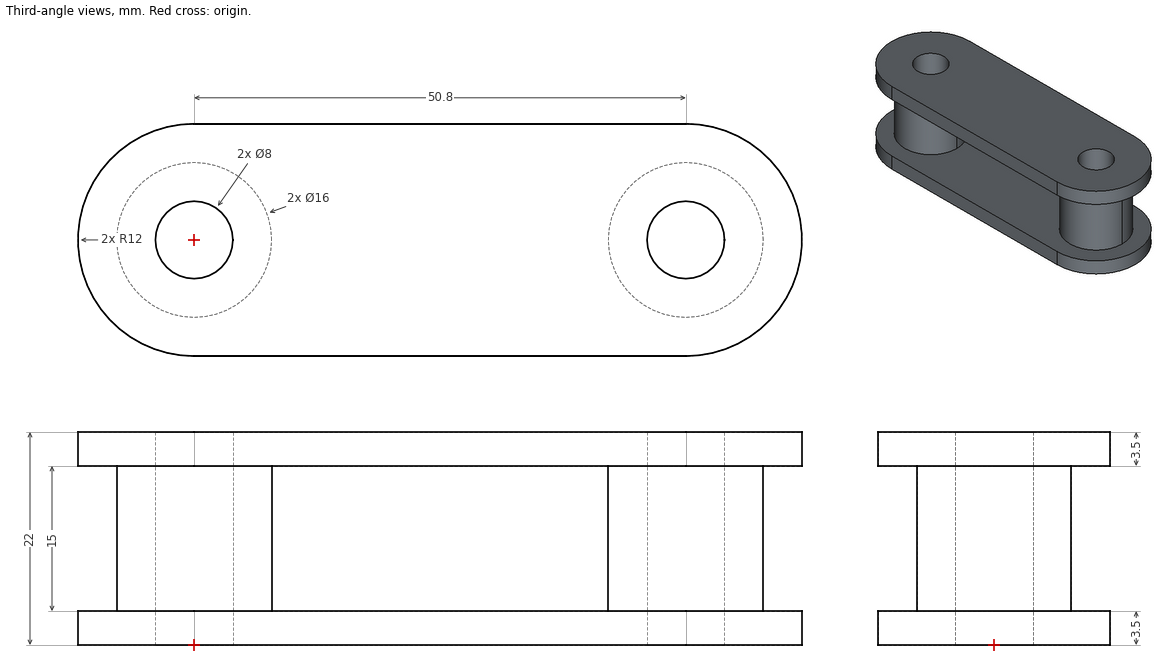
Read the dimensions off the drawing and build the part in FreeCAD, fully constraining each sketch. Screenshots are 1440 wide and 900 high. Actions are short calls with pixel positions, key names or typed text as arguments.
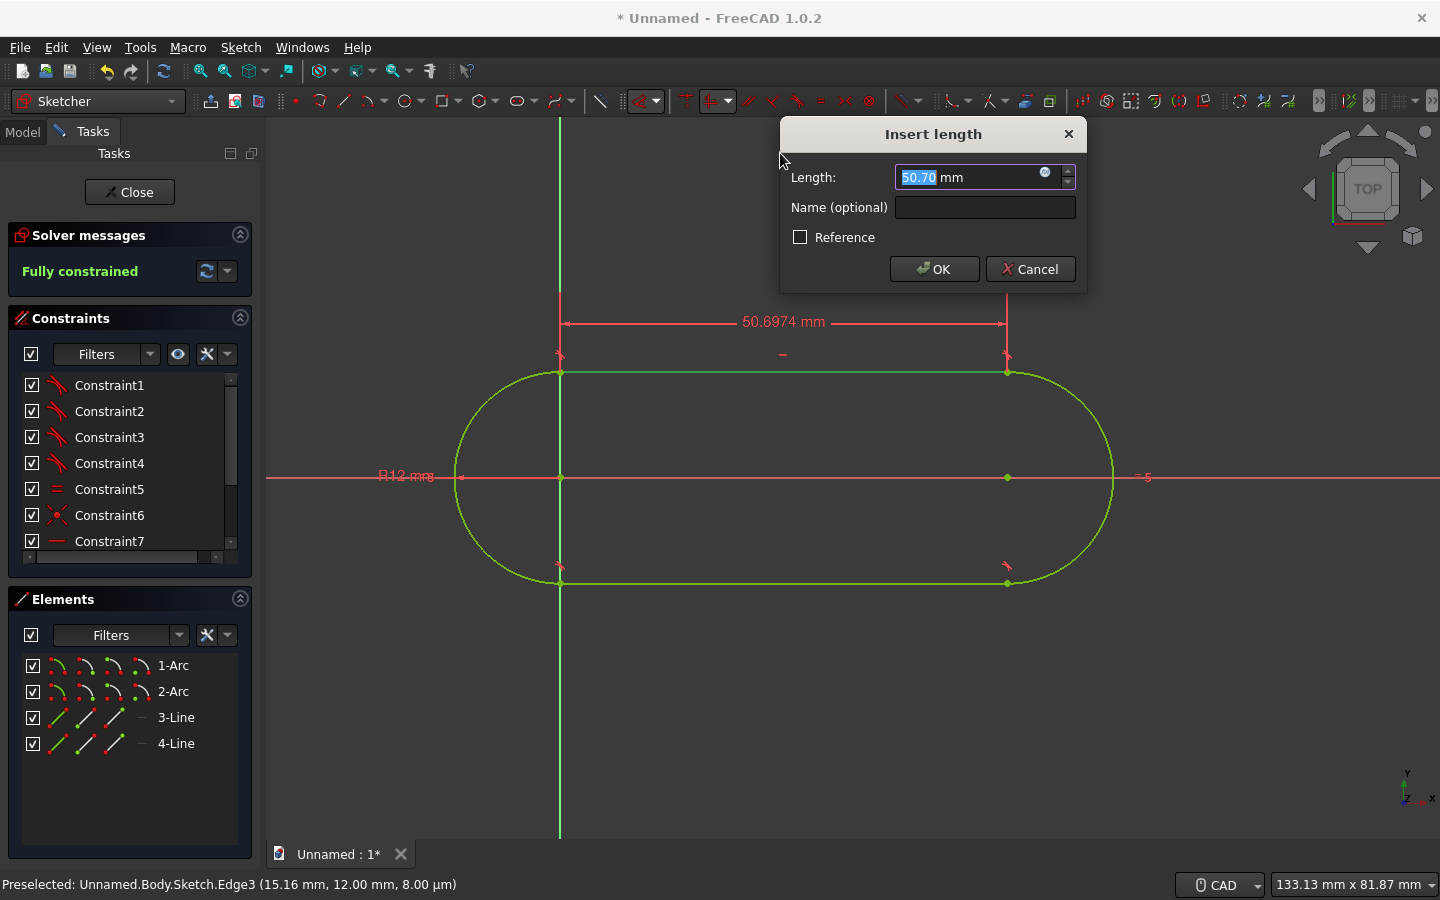
text(50.8)
key(Return)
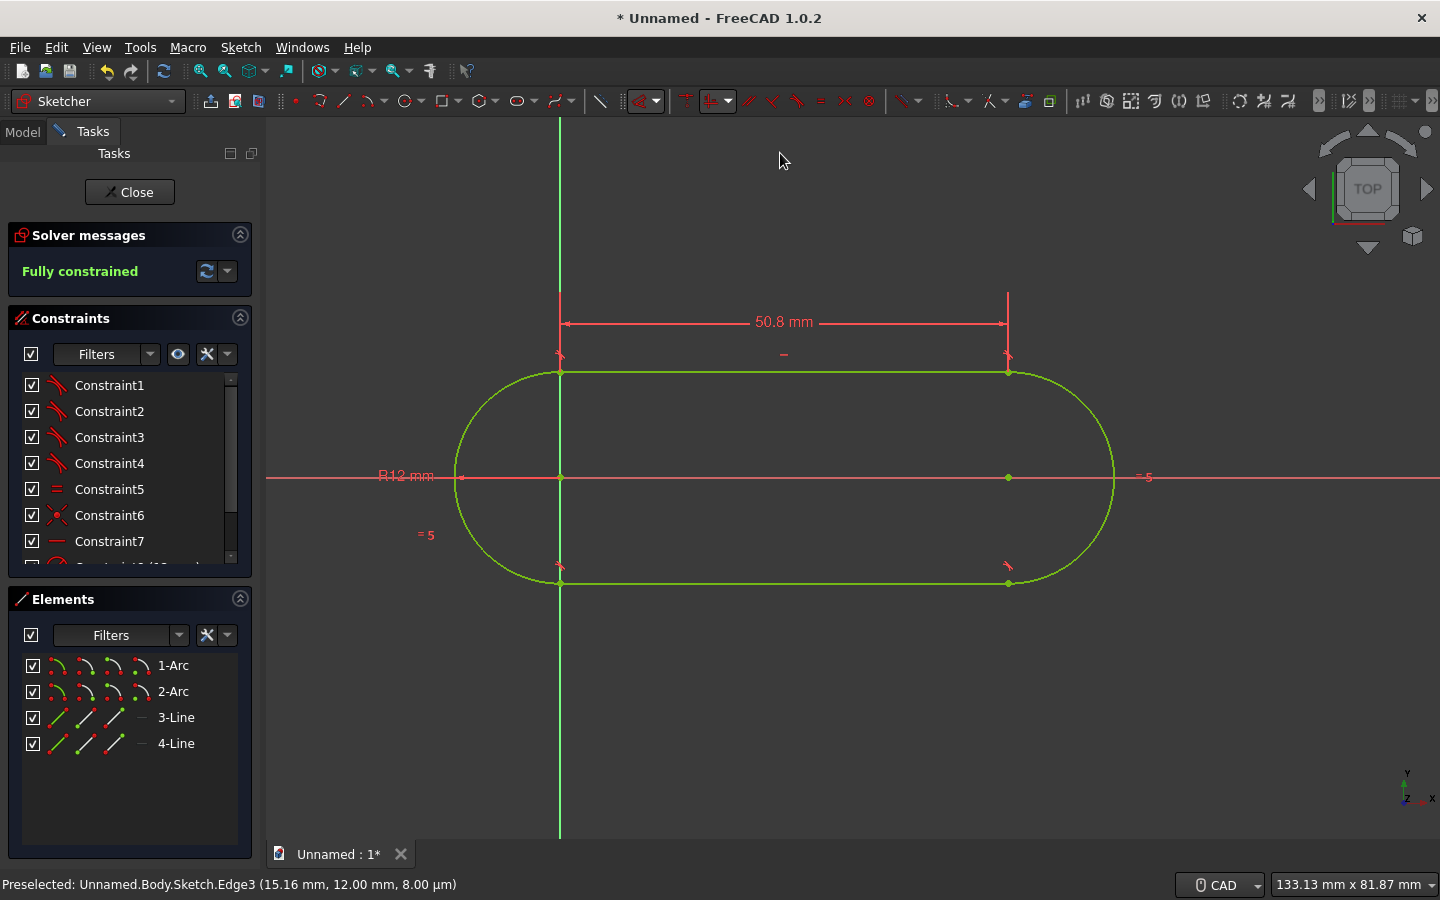
click(130, 192)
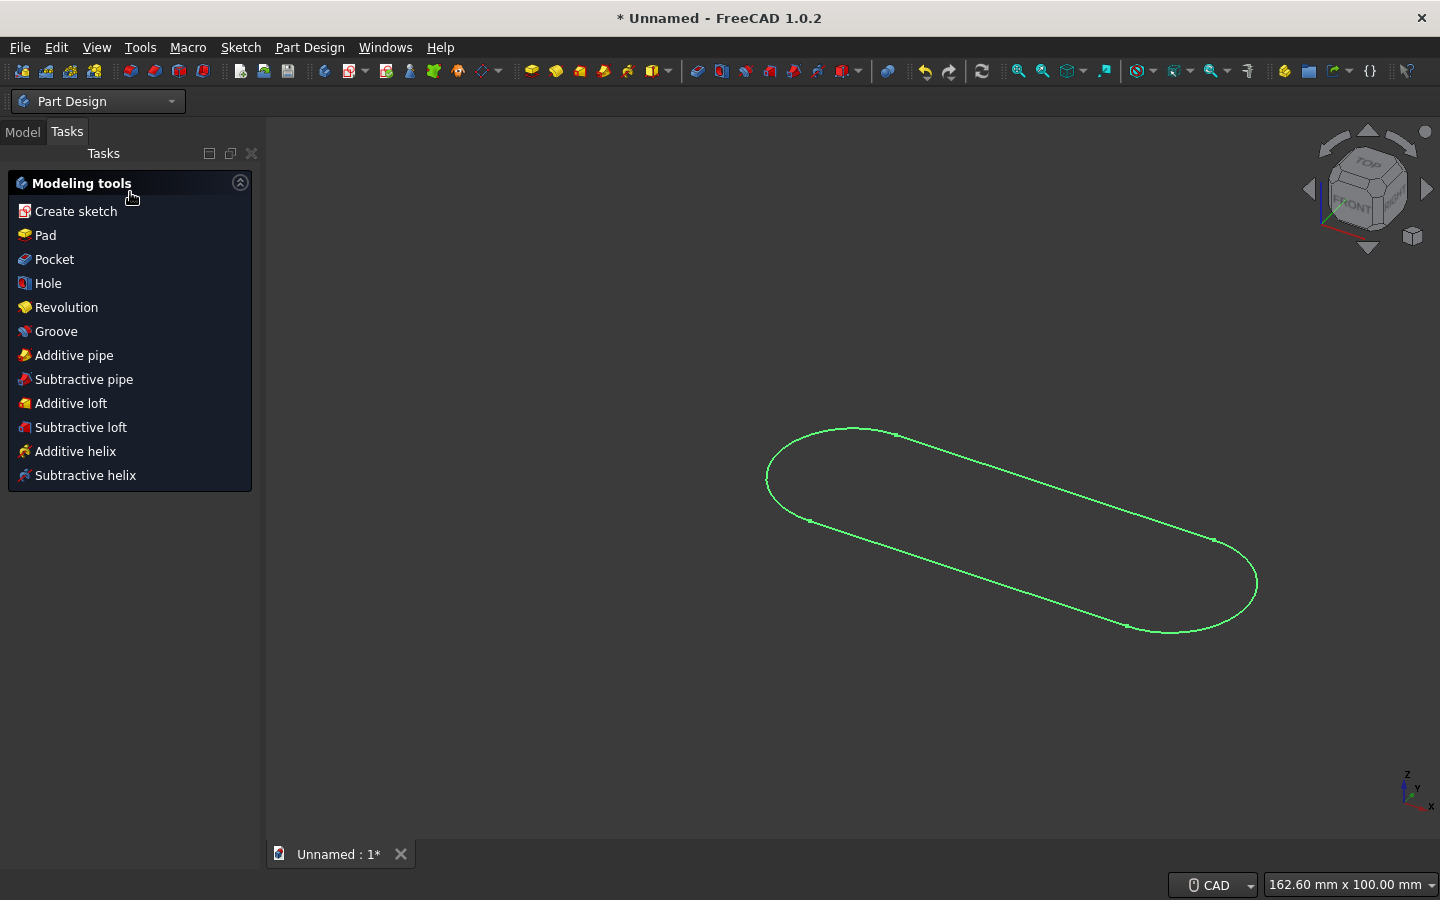
click(532, 72)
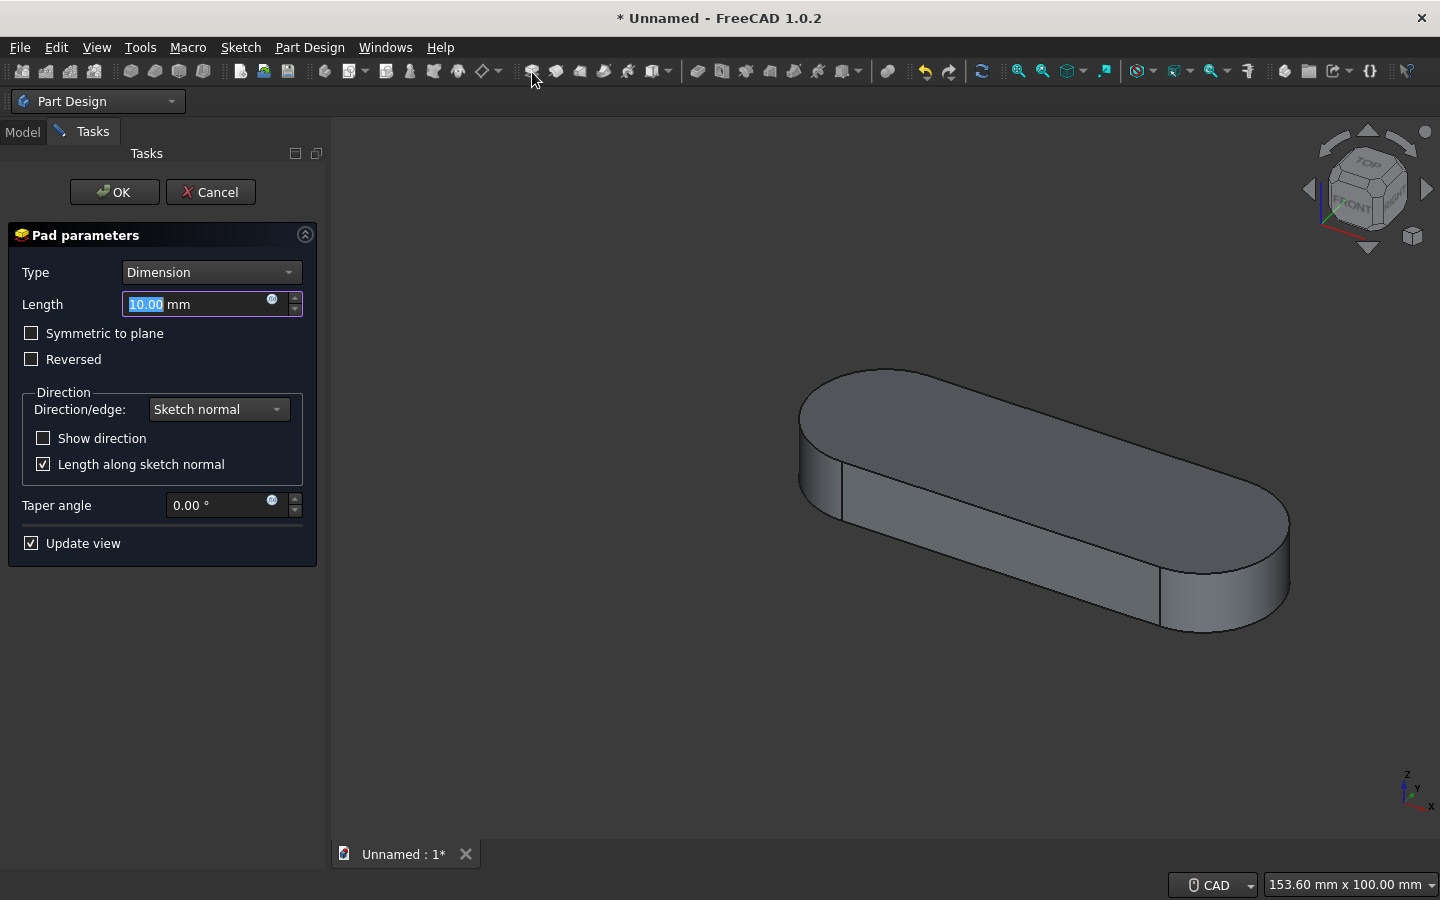
text(3.5)
key(Tab)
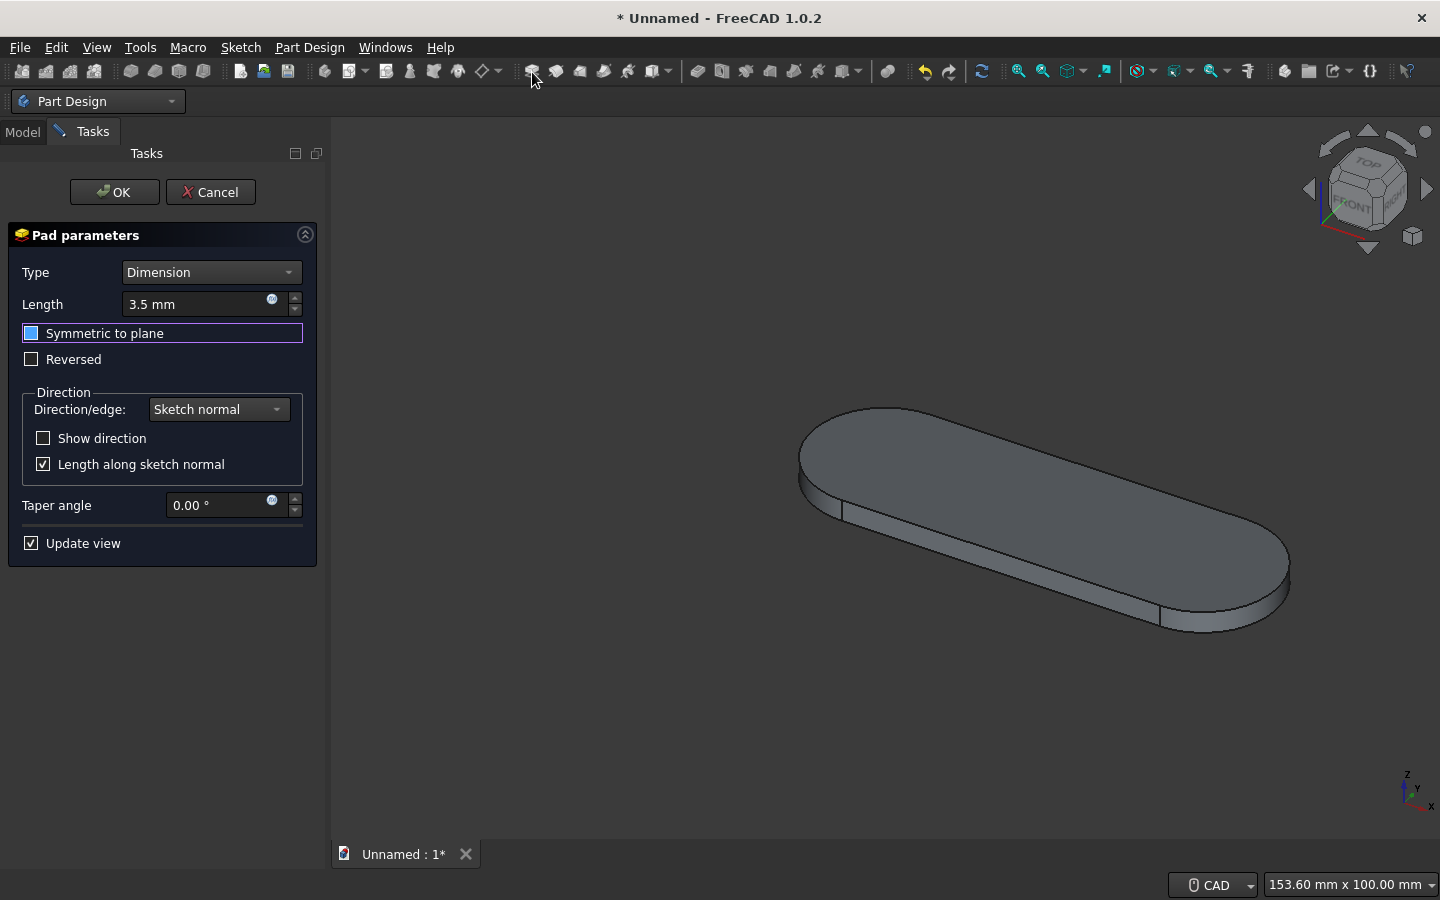
click(115, 192)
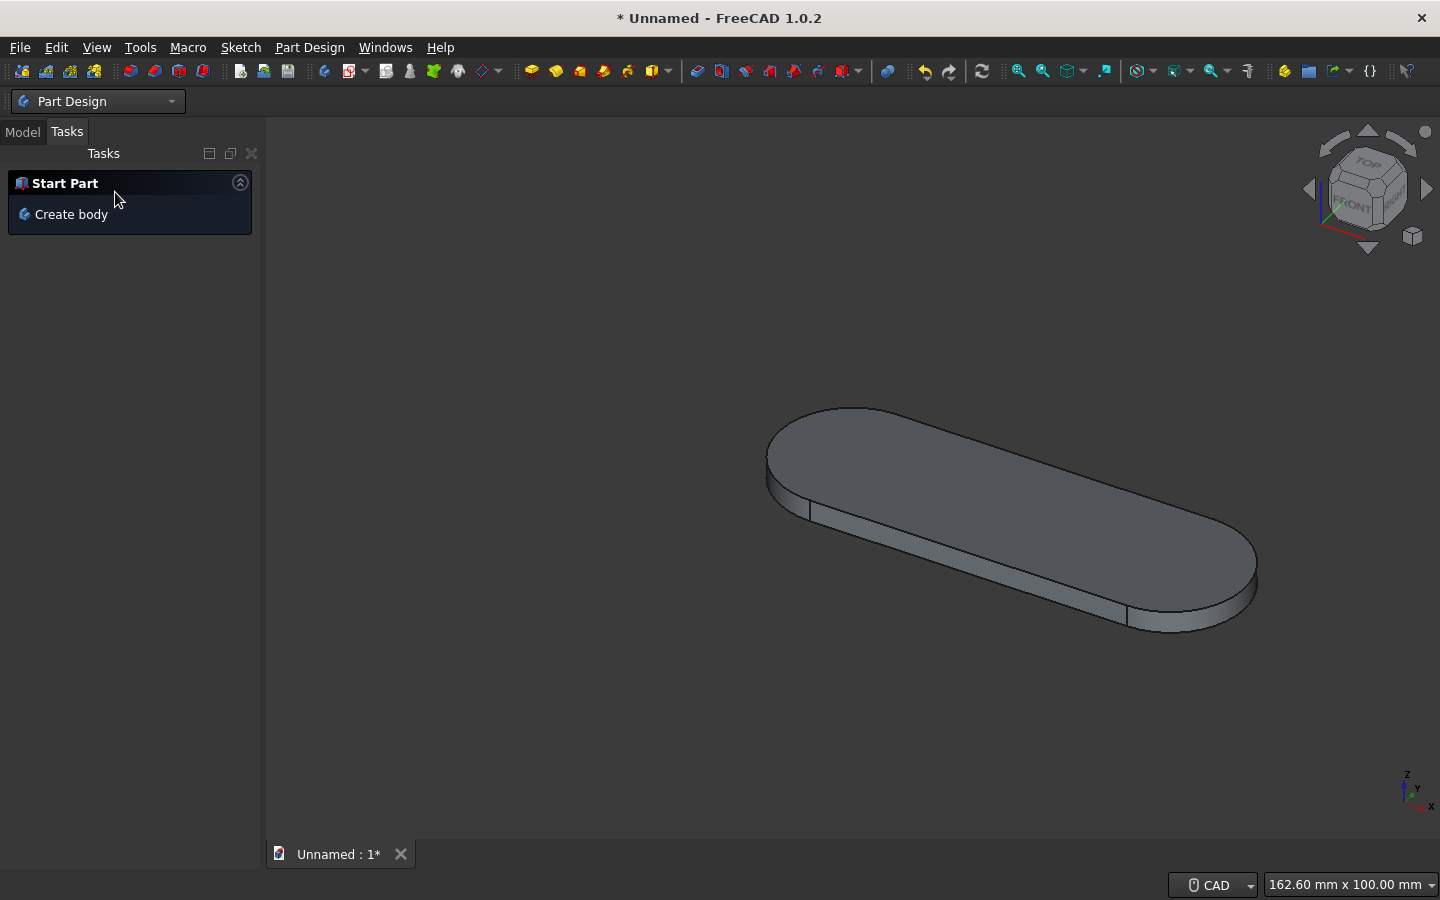
click(1145, 553)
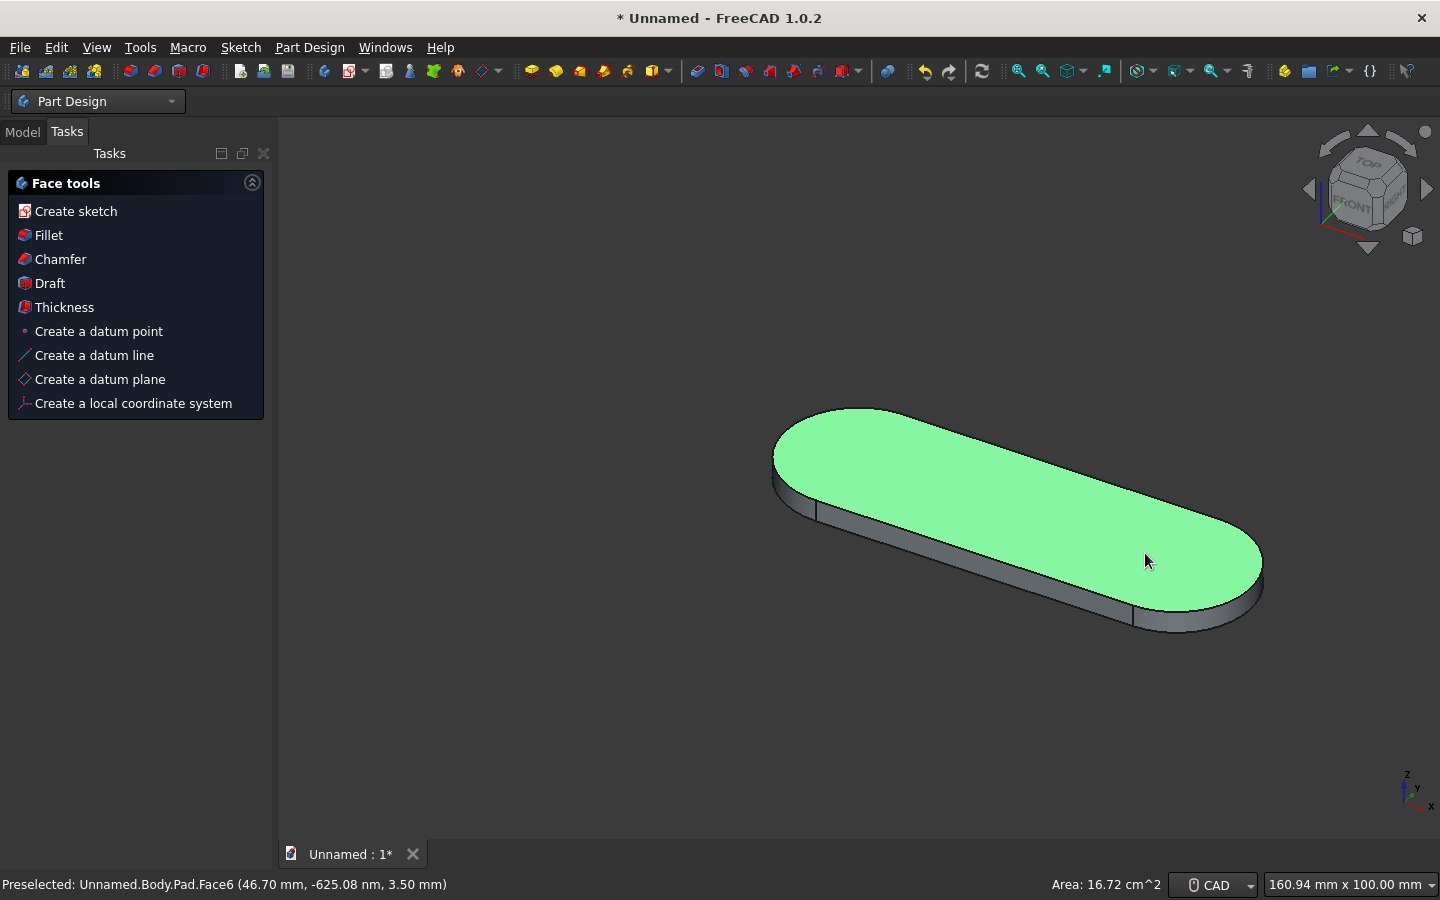
click(350, 72)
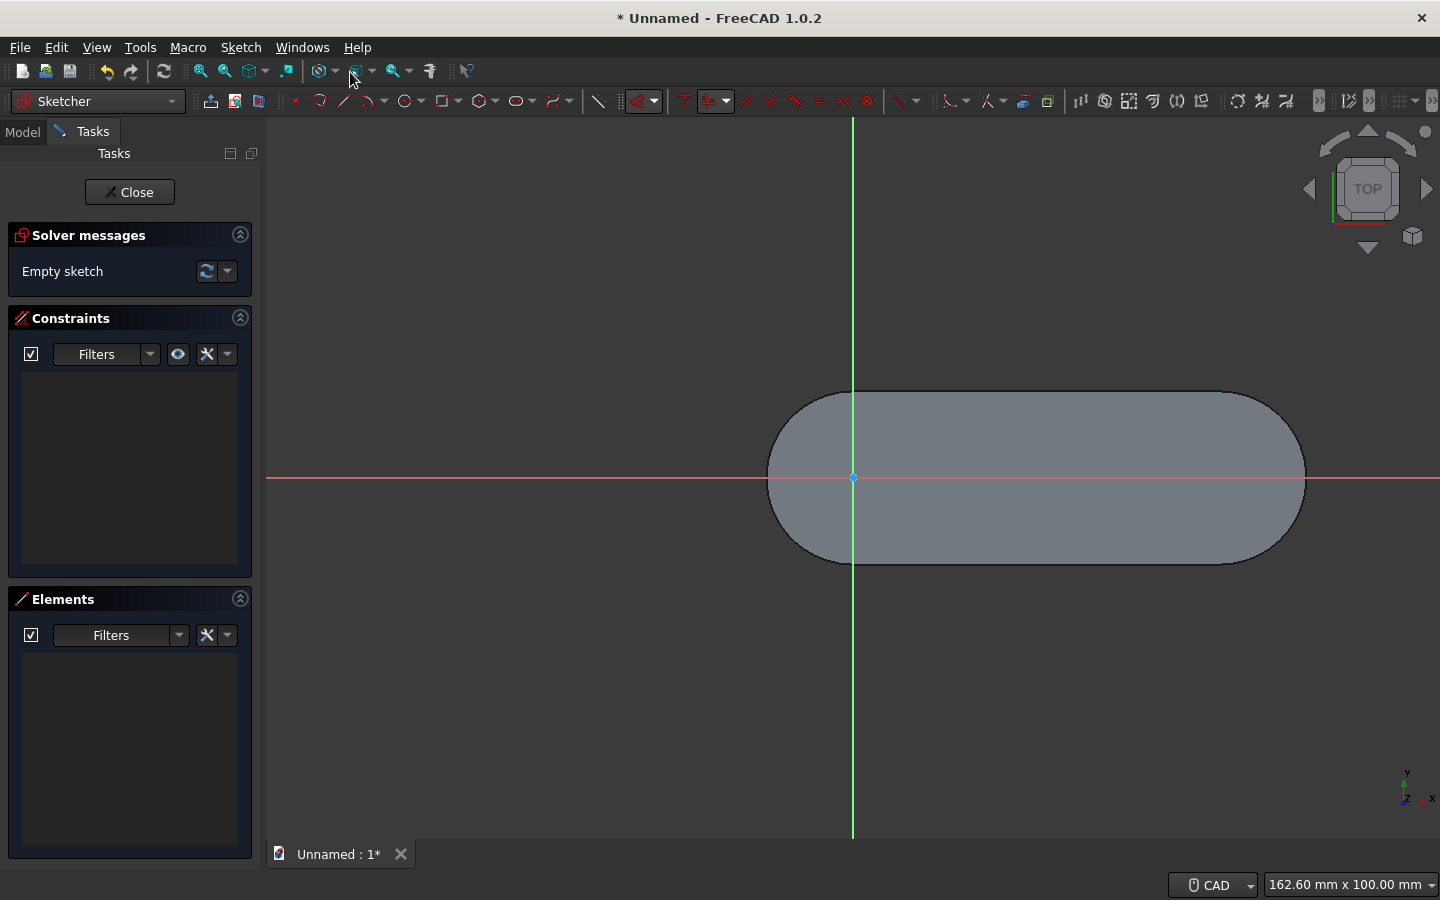
scroll(294, 478, down, 1)